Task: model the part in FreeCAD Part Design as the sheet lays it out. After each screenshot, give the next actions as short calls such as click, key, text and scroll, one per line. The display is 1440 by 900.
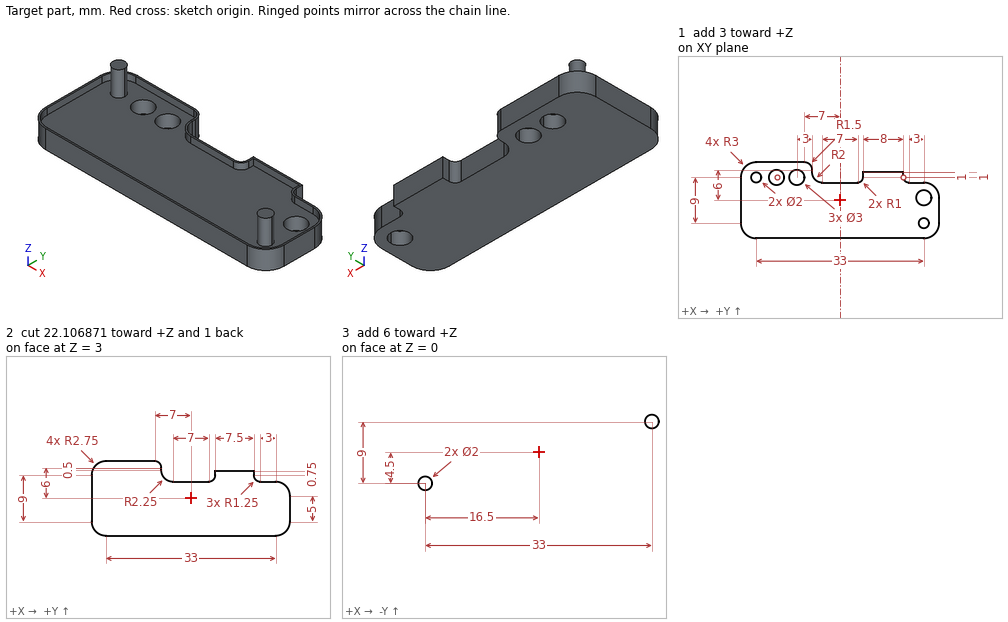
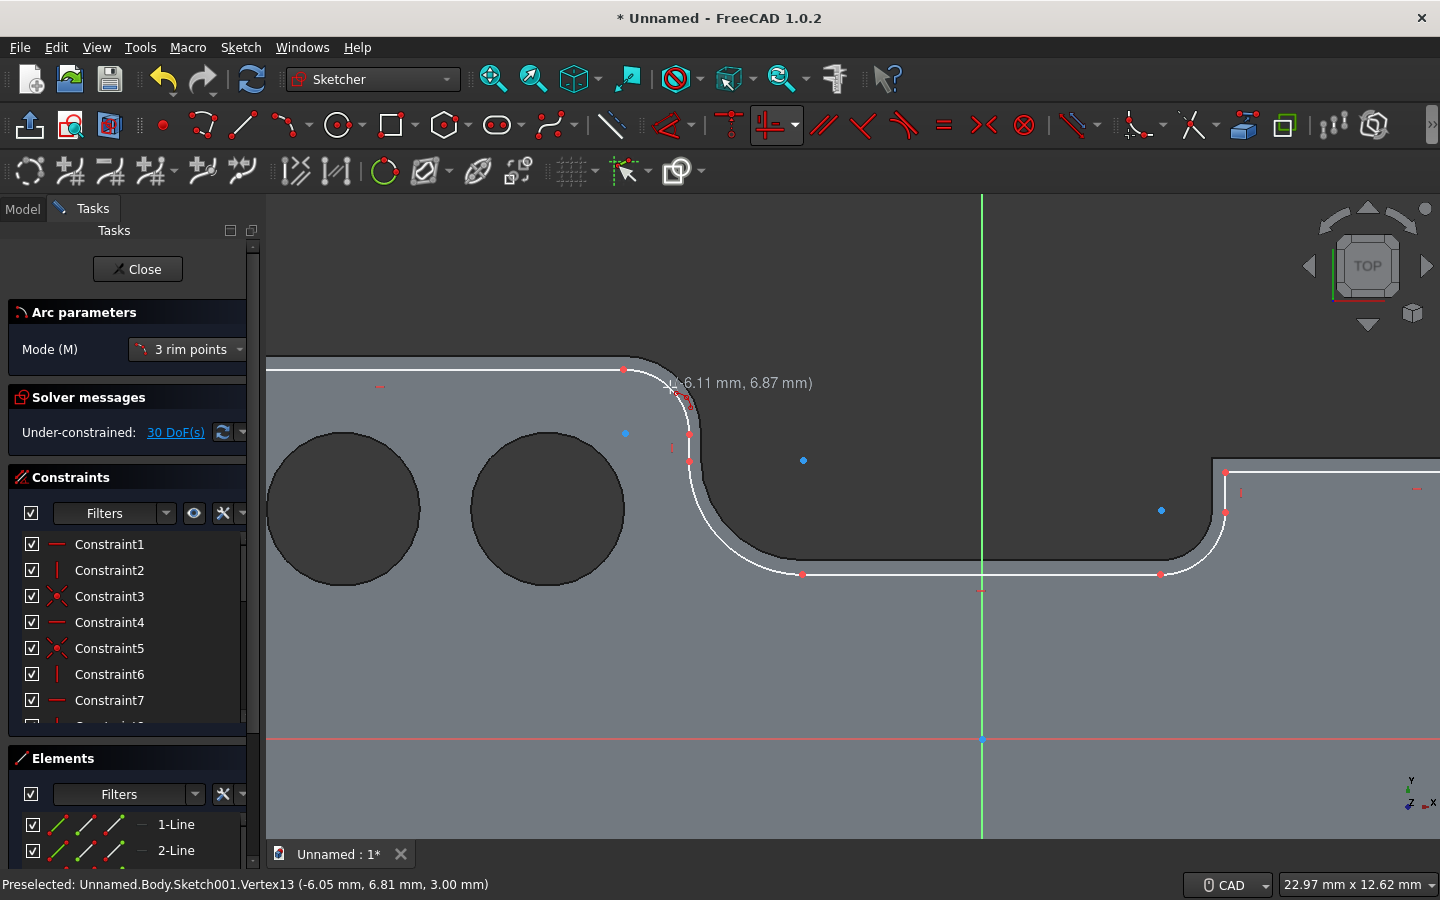
scroll(669, 387, down, 5)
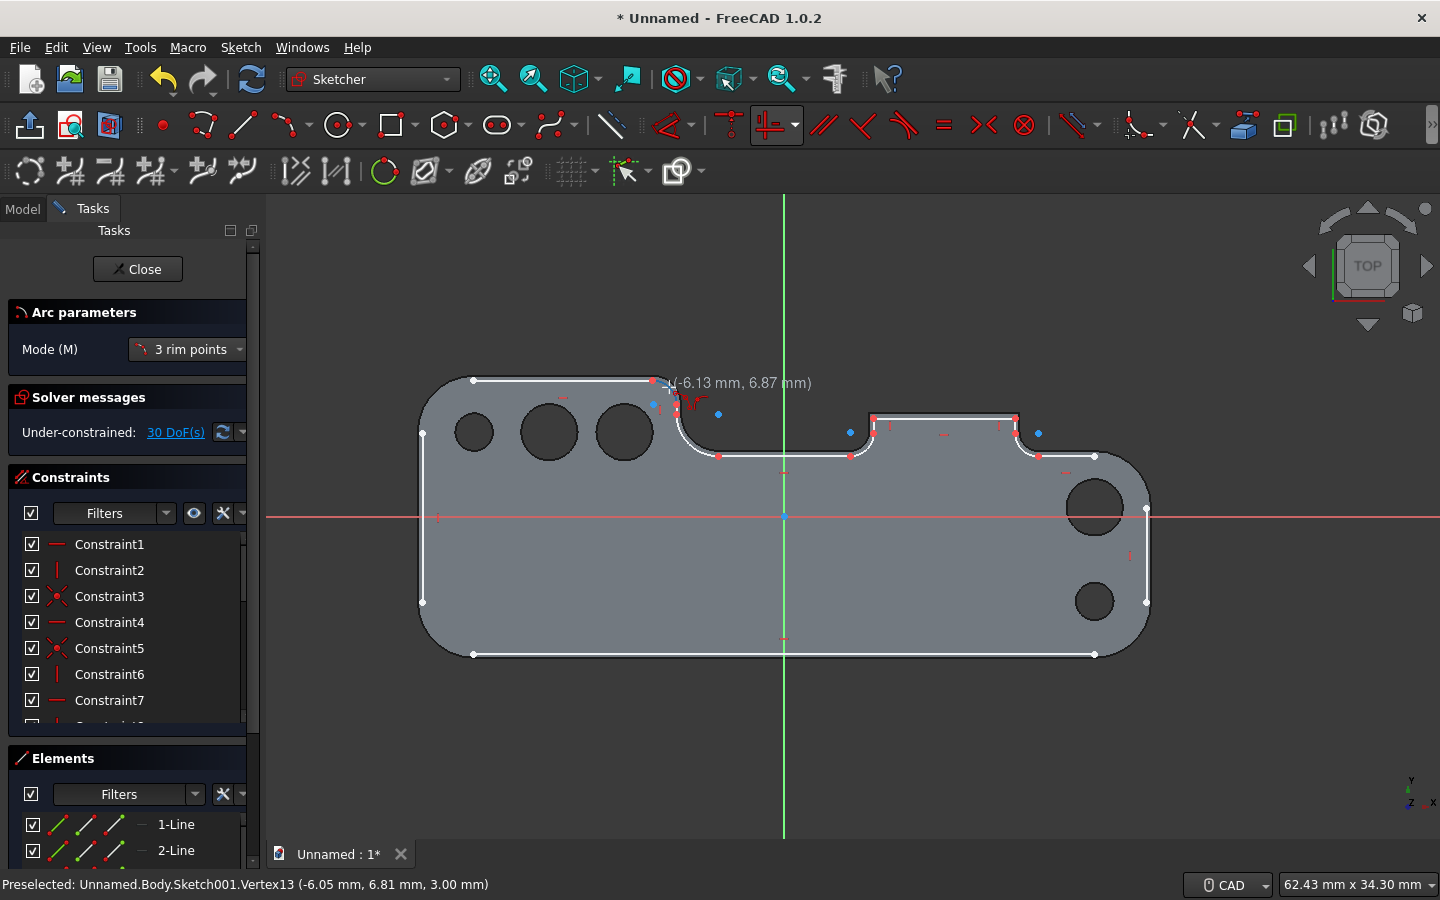
click(474, 381)
click(423, 433)
click(438, 396)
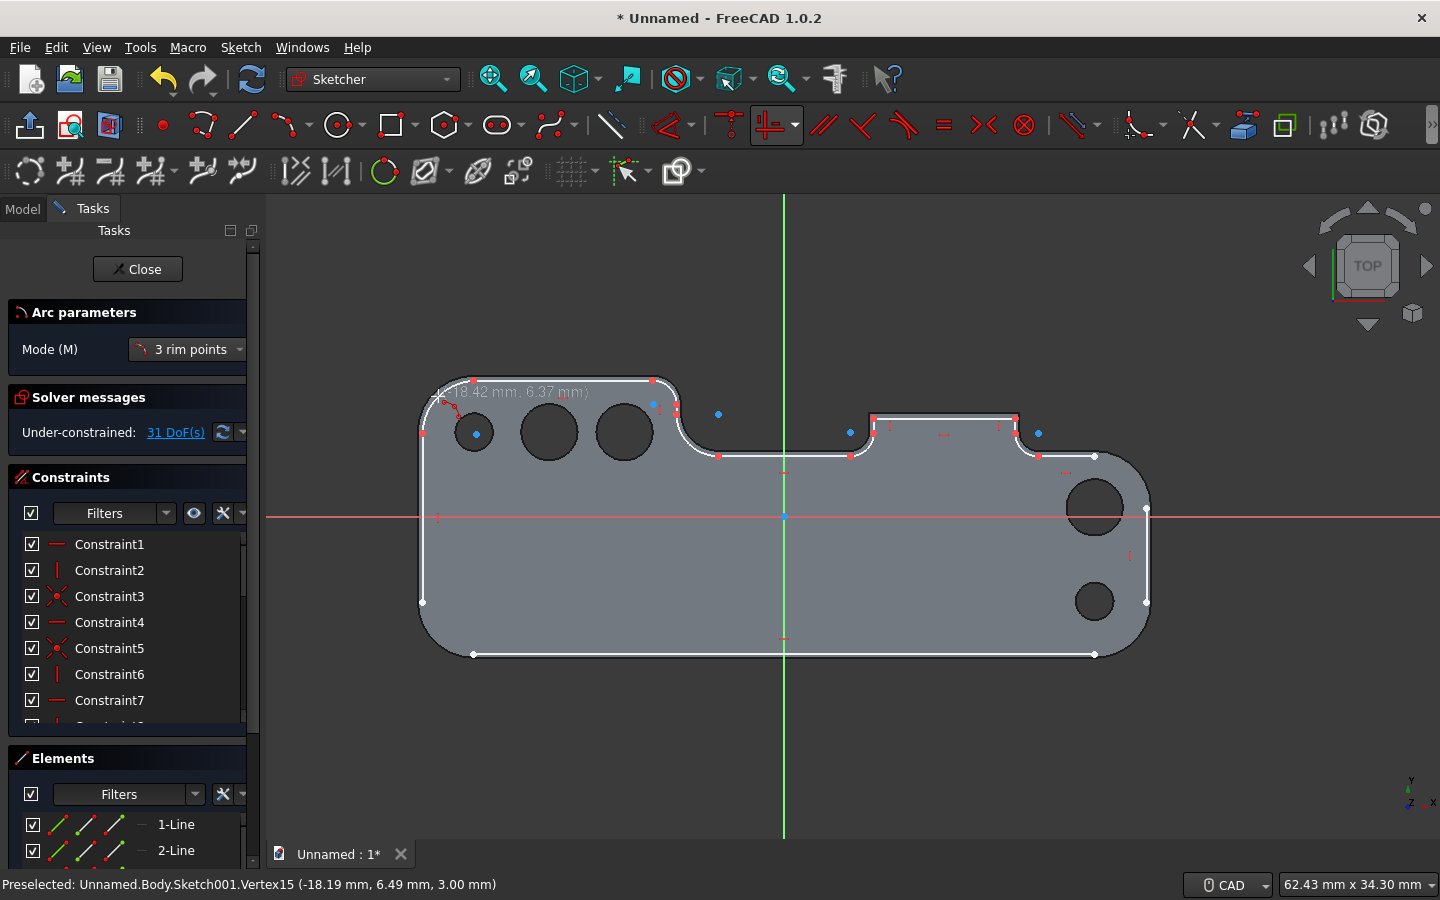
click(423, 602)
click(474, 654)
click(438, 638)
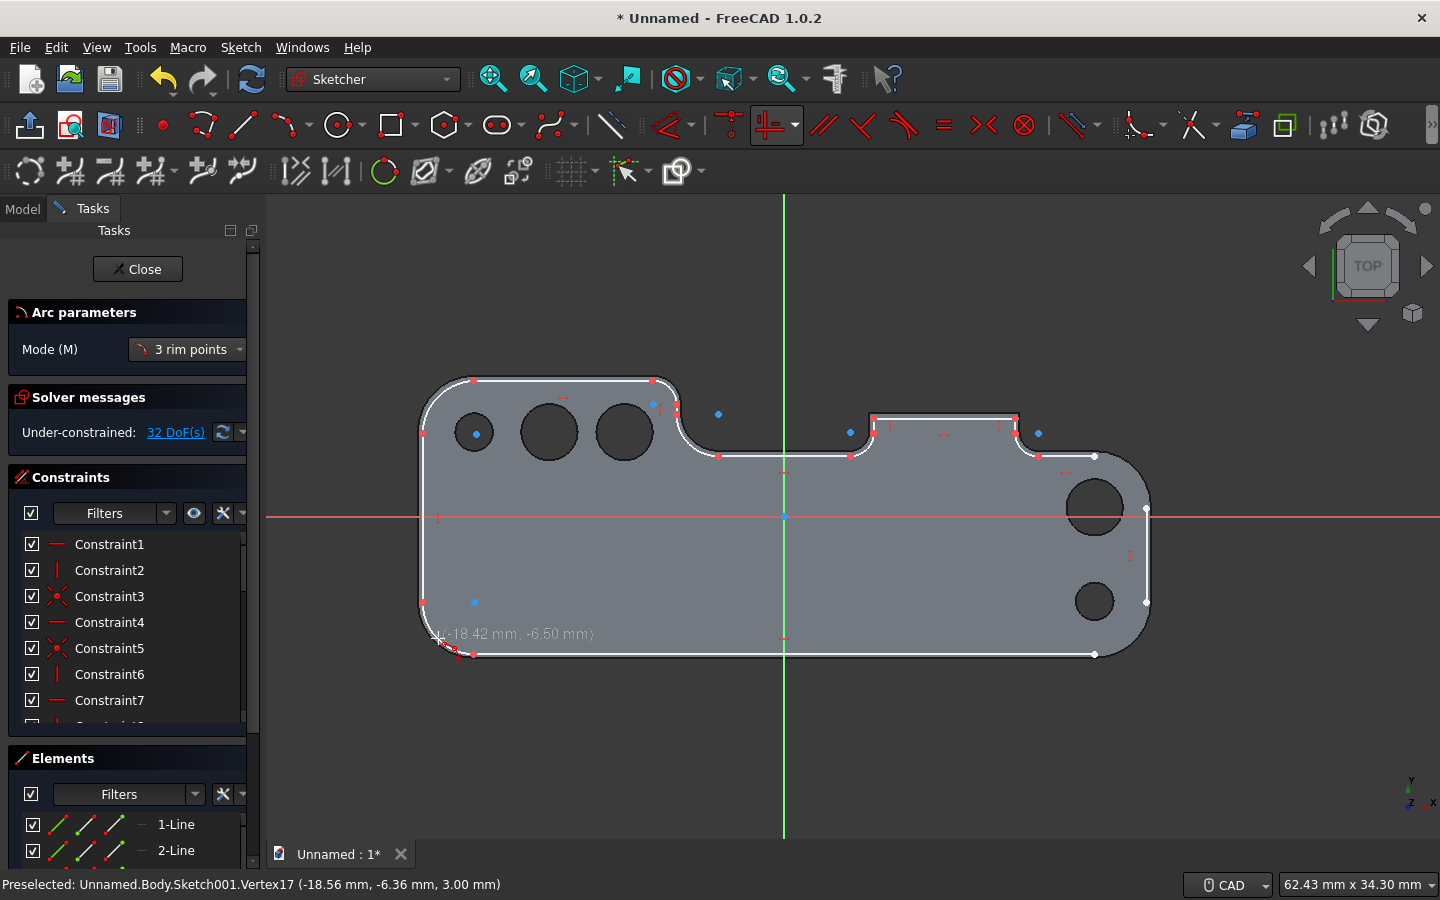
click(1095, 654)
click(1147, 602)
click(1131, 638)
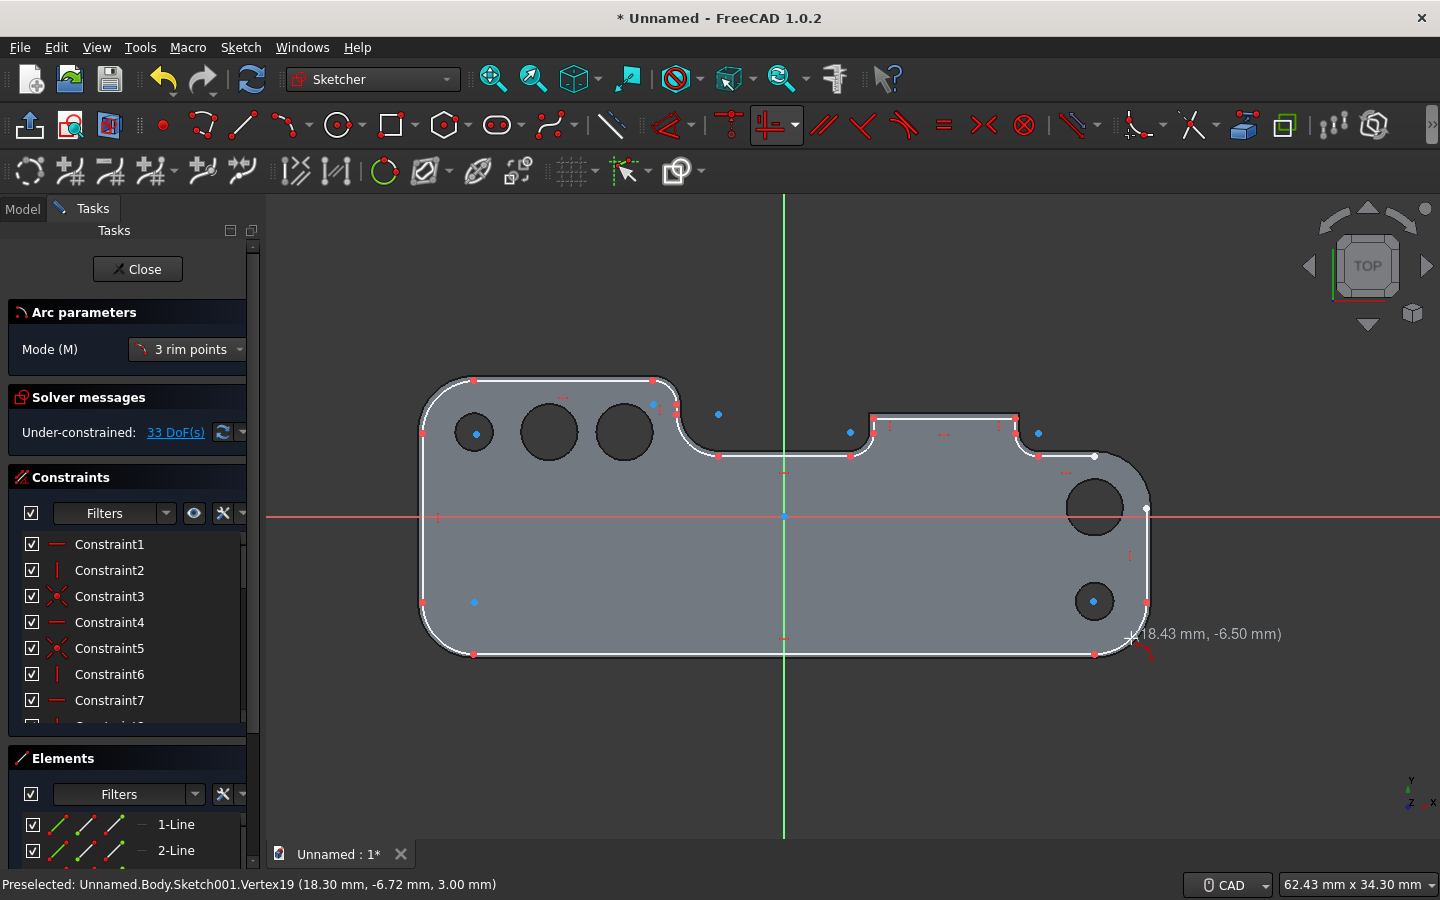
scroll(1146, 507, up, 3)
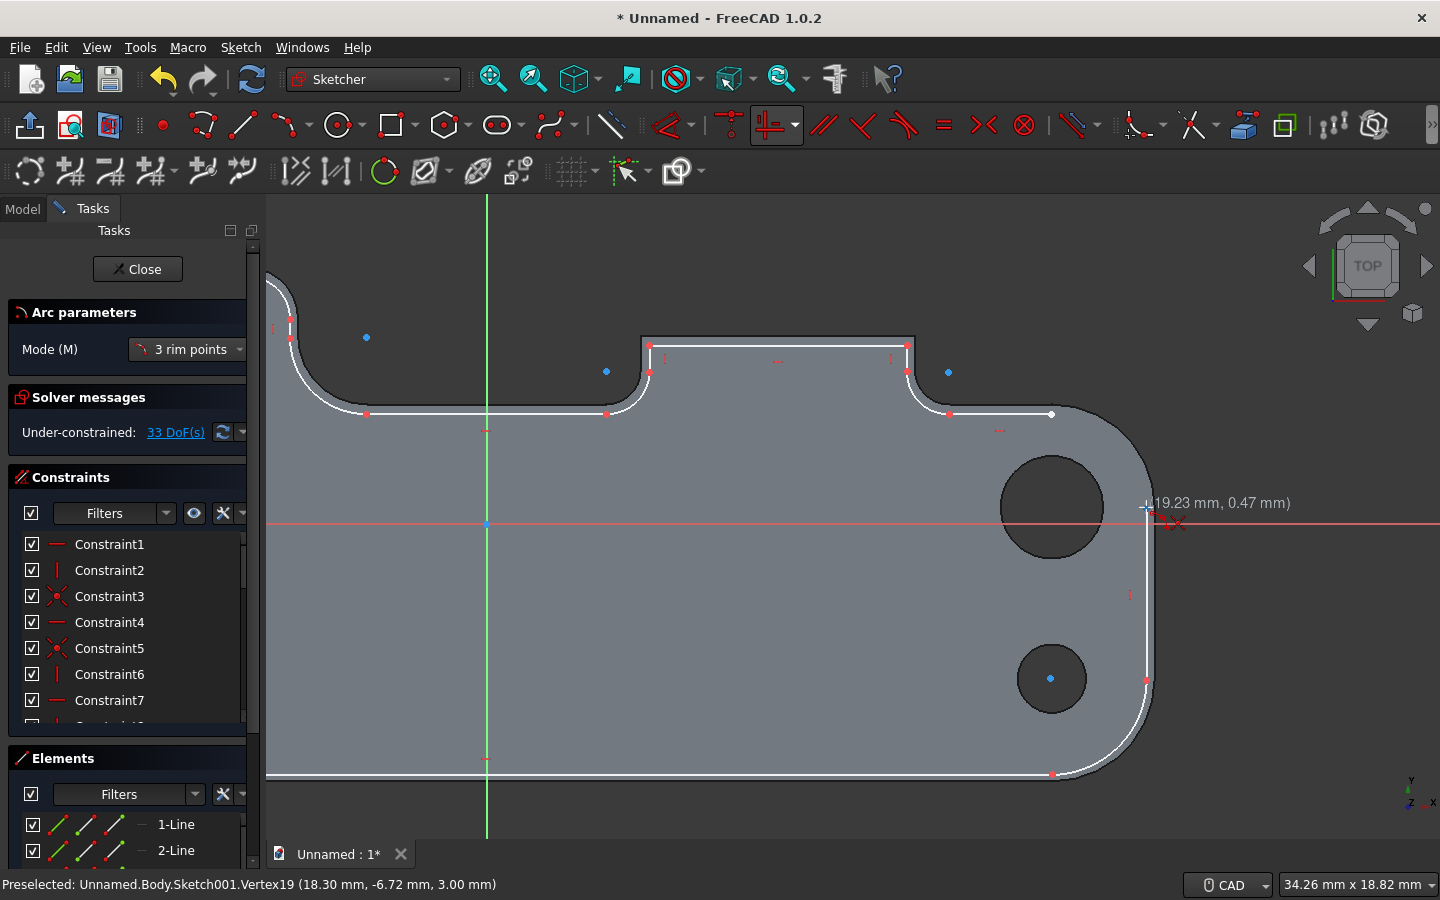
click(1147, 508)
click(1052, 414)
click(1119, 441)
key(Escape)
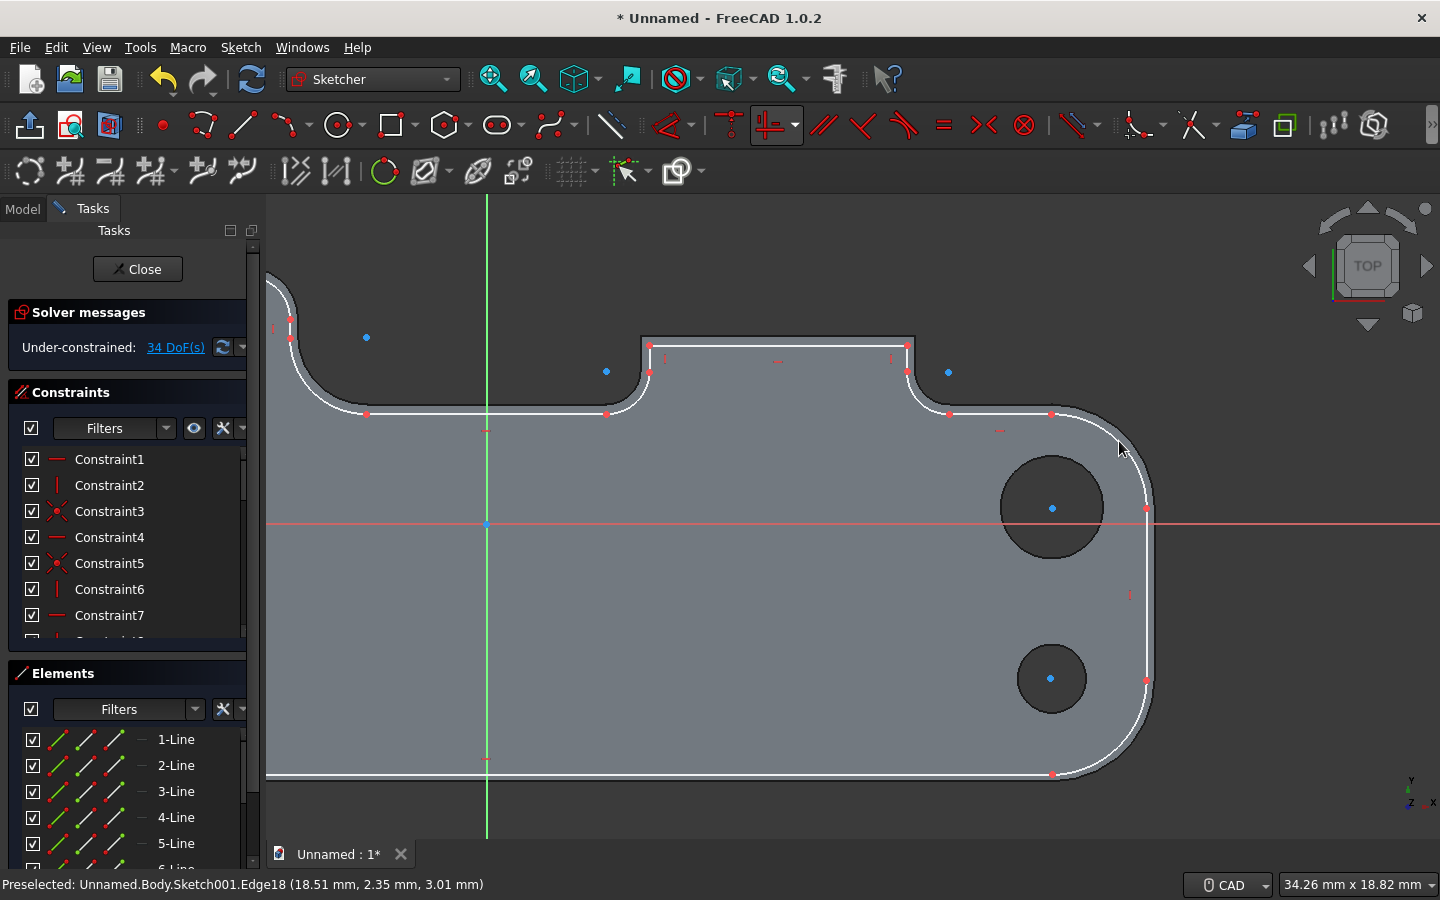
click(1021, 414)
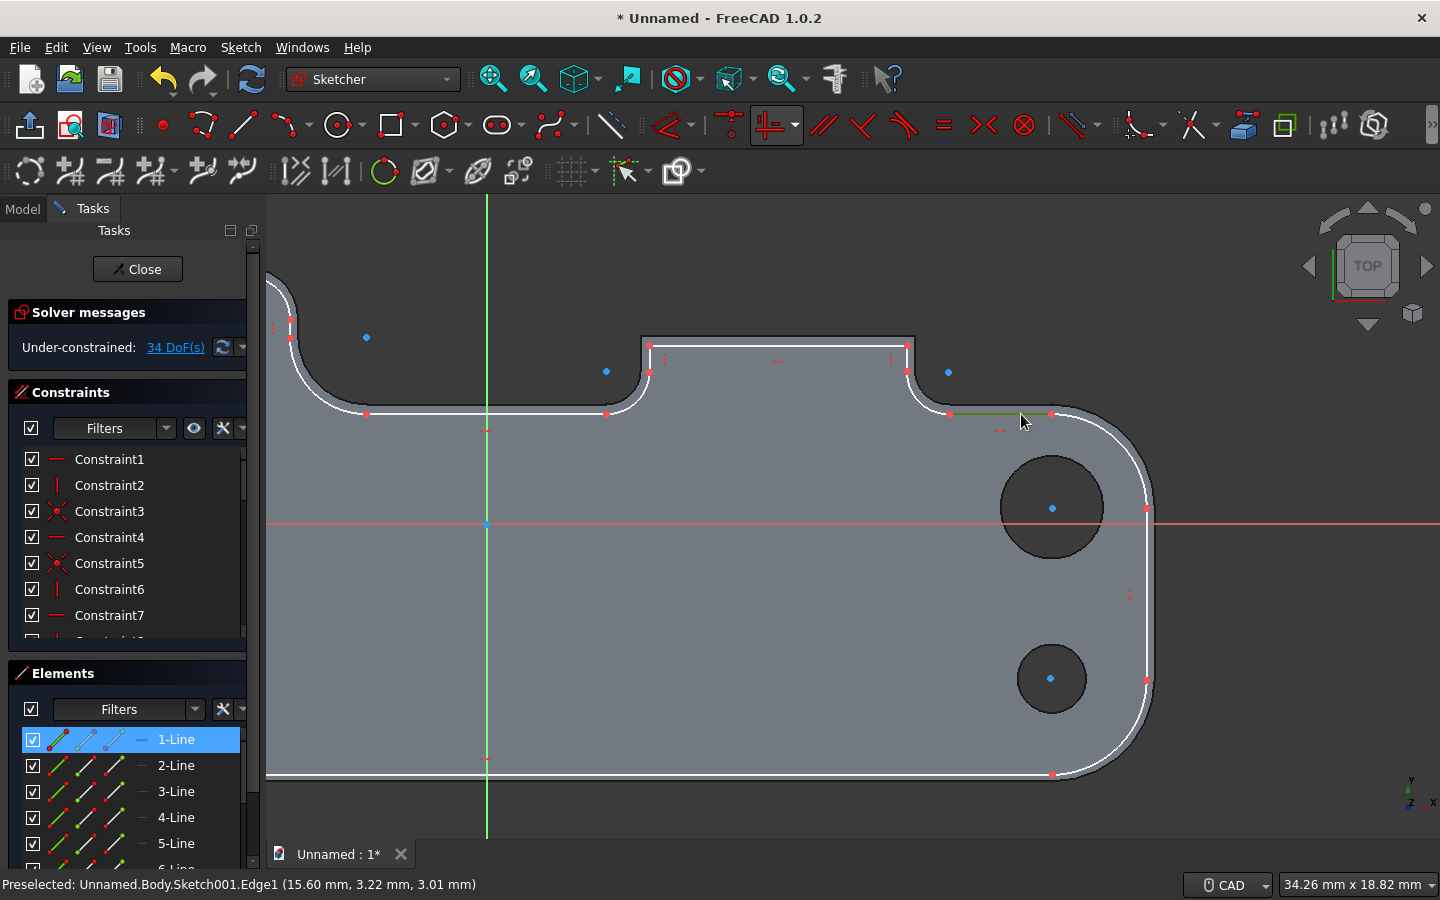
click(912, 391)